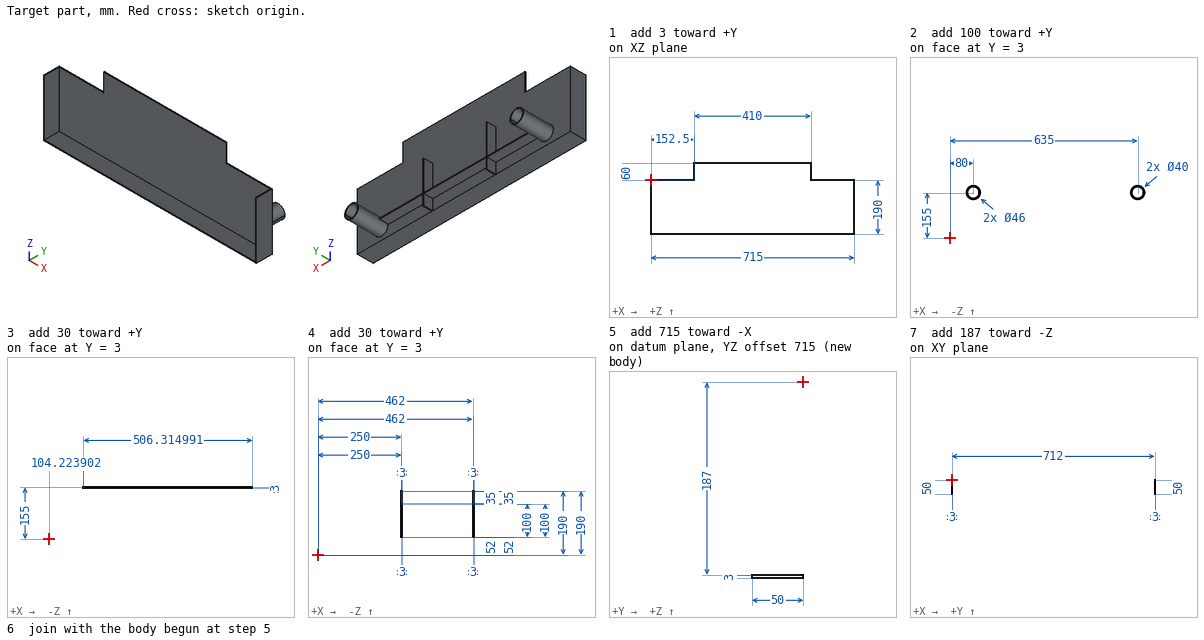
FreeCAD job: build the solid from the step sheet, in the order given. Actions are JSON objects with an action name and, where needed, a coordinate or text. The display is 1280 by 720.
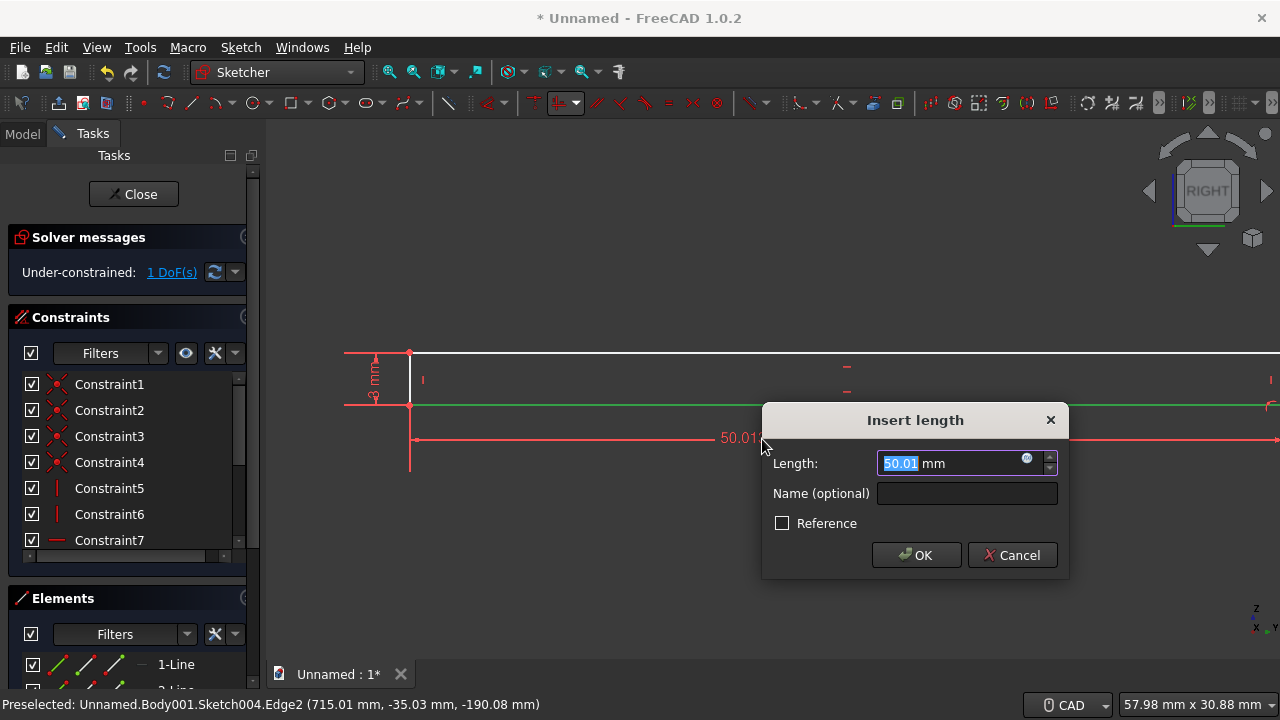
{"action": "type", "text": "50"}
{"action": "key", "text": "Return"}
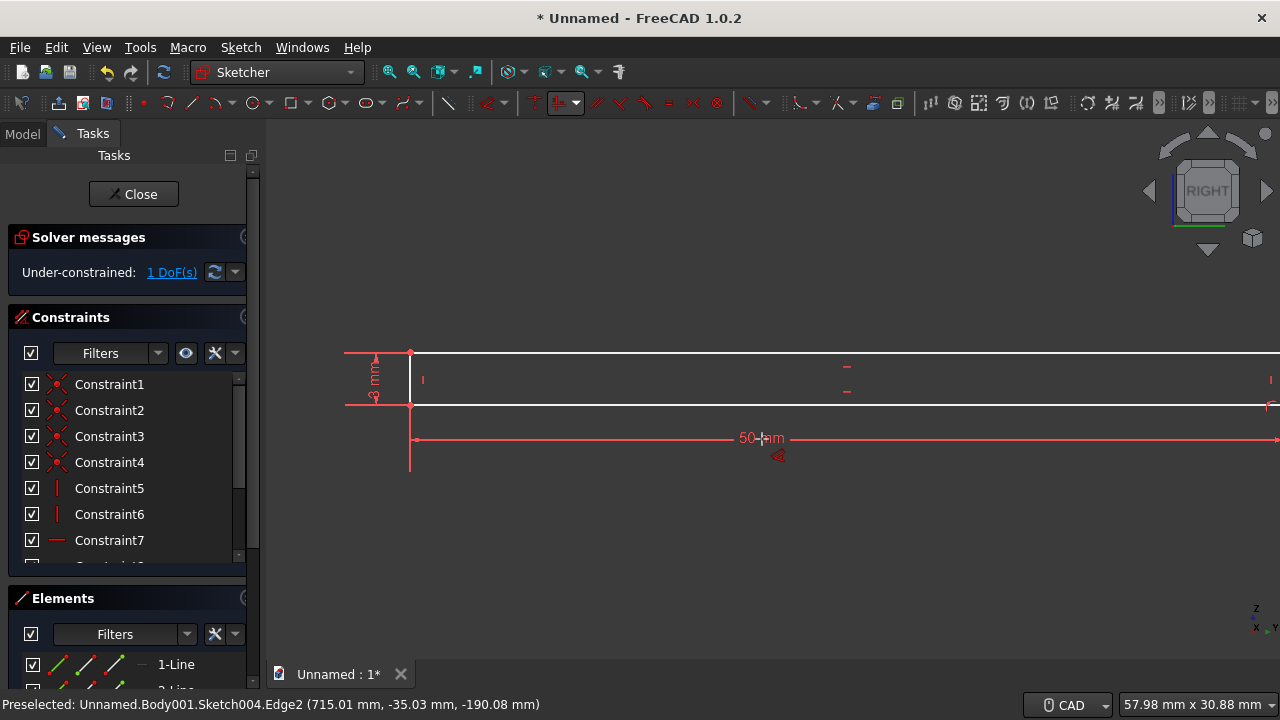
{"action": "left_click", "coordinate": [410, 353]}
{"action": "left_click", "coordinate": [376, 250]}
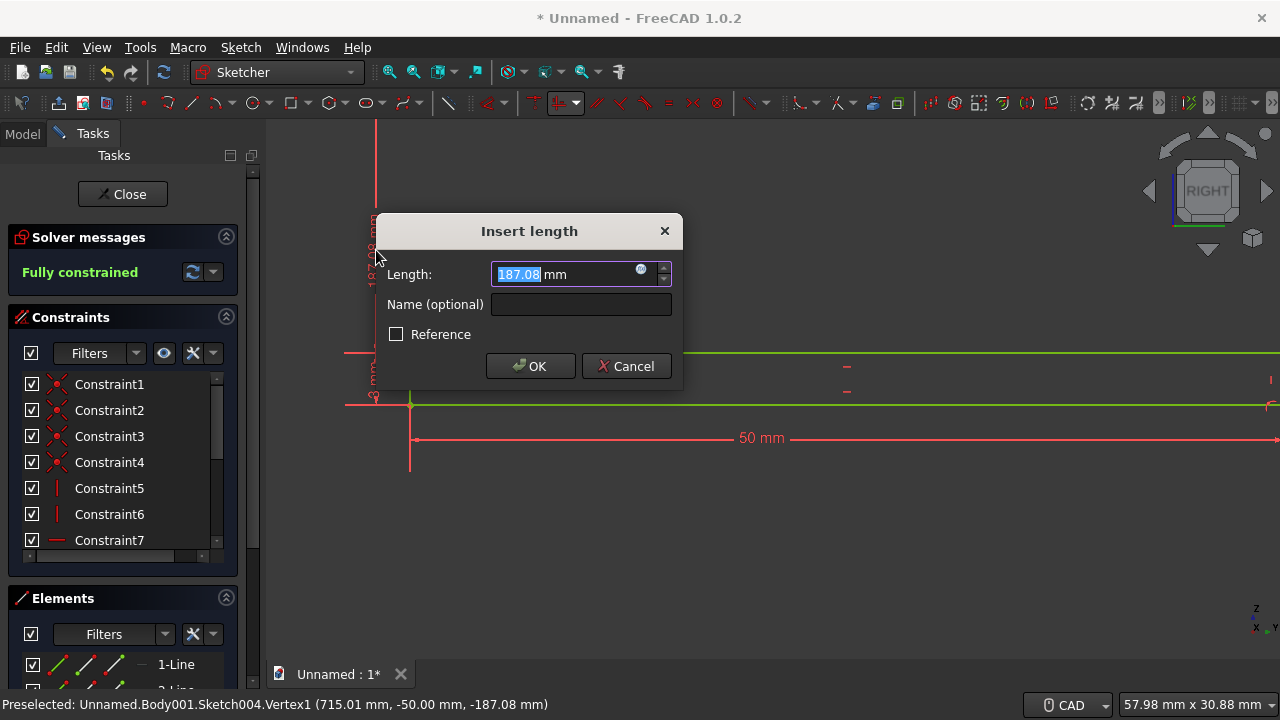
{"action": "type", "text": "187"}
{"action": "key", "text": "Return"}
{"action": "key", "text": "Escape"}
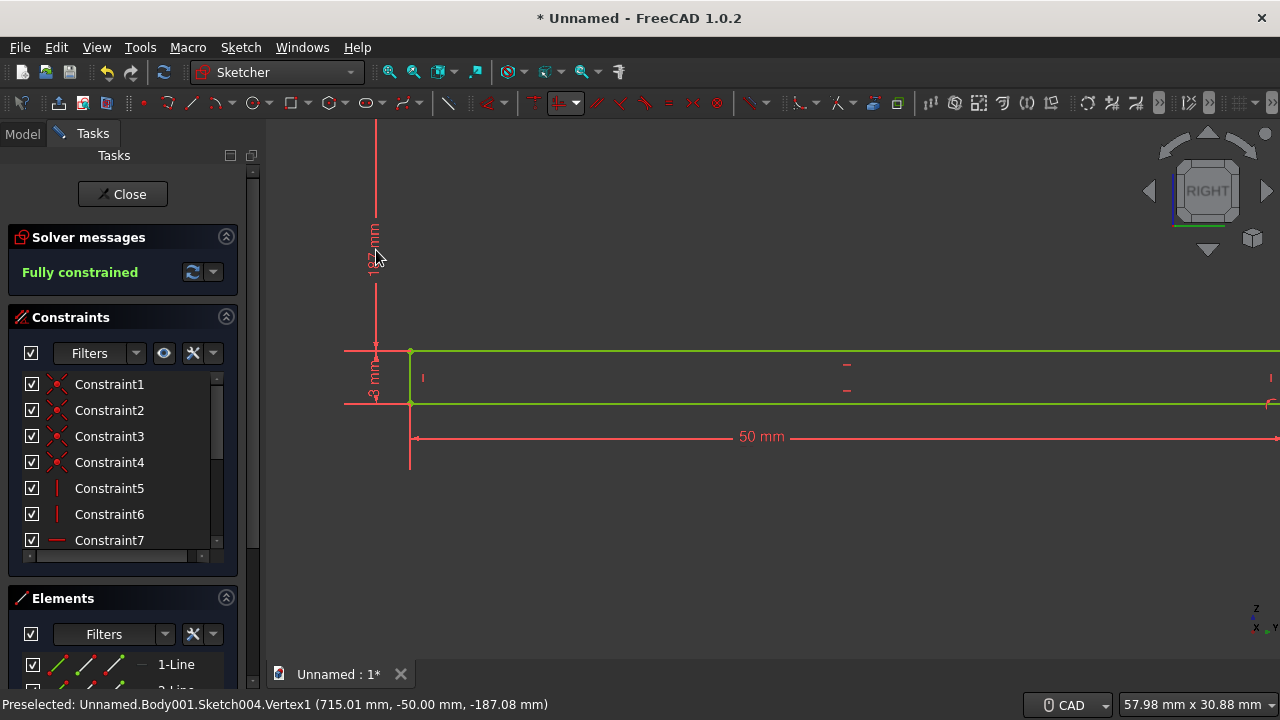
{"action": "left_click", "coordinate": [123, 194]}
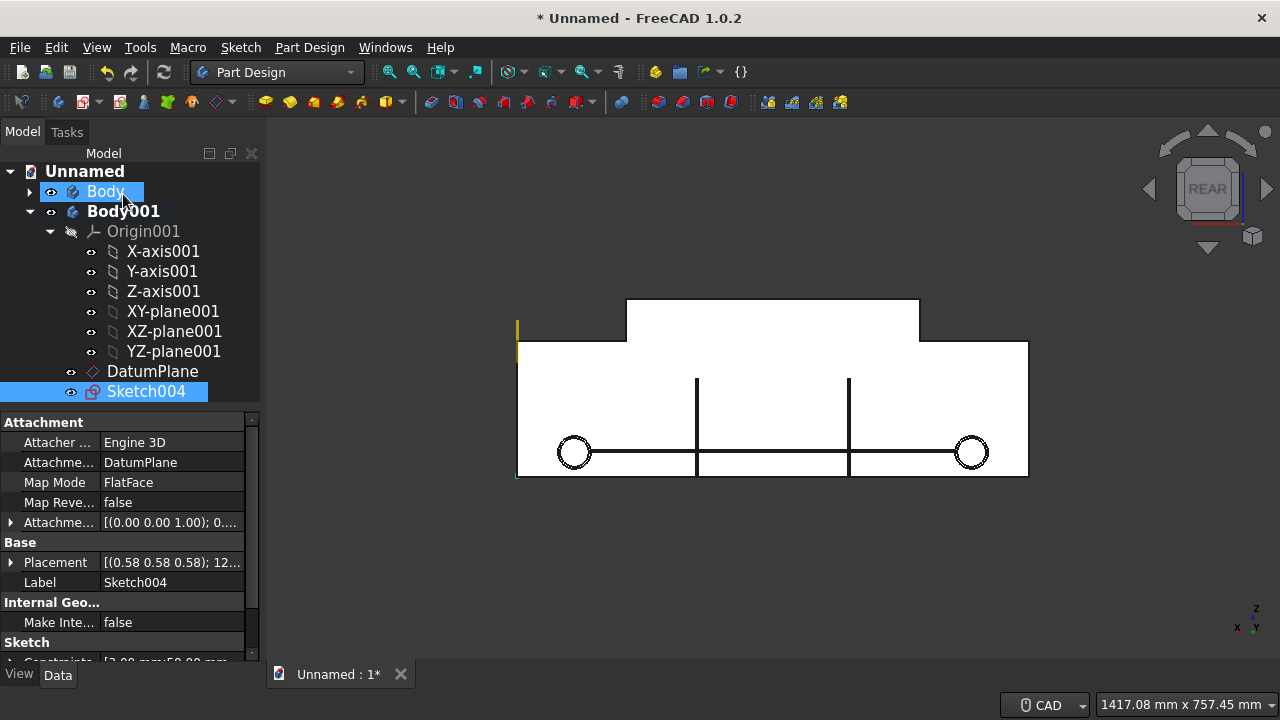
{"action": "left_click", "coordinate": [266, 102]}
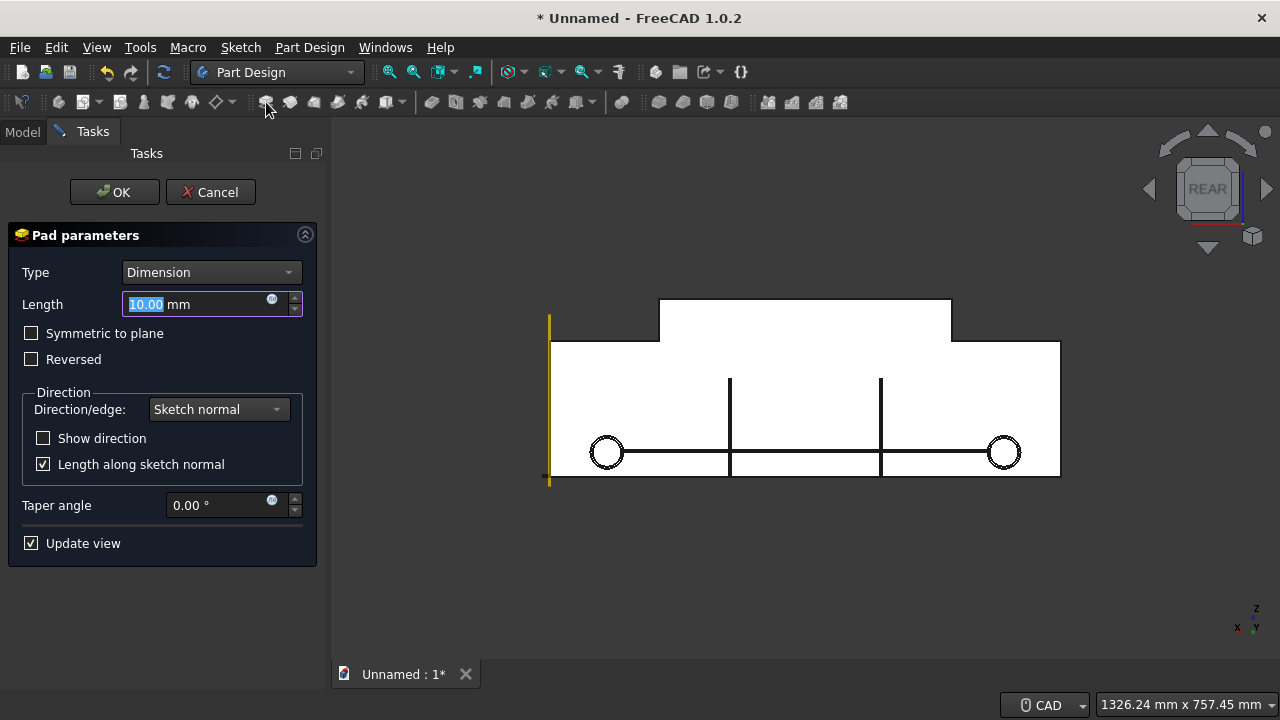
{"action": "type", "text": "715"}
{"action": "key", "text": "Tab"}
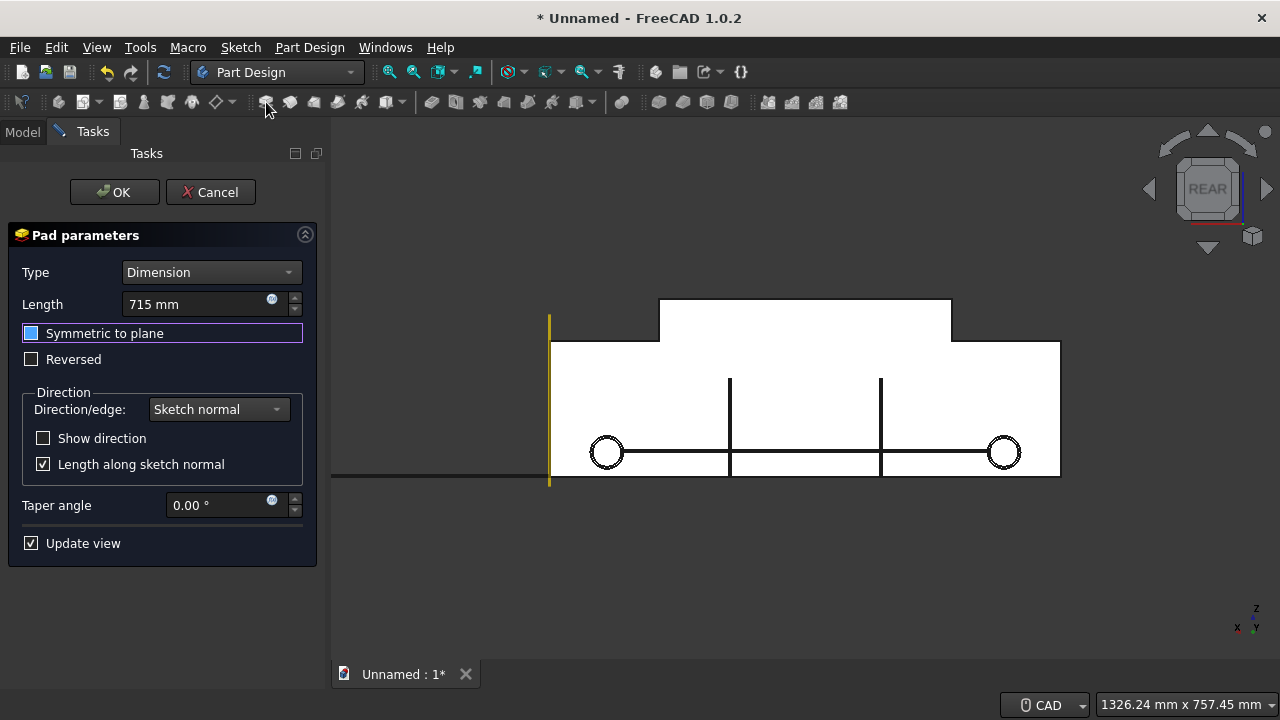
{"action": "left_click", "coordinate": [30, 359]}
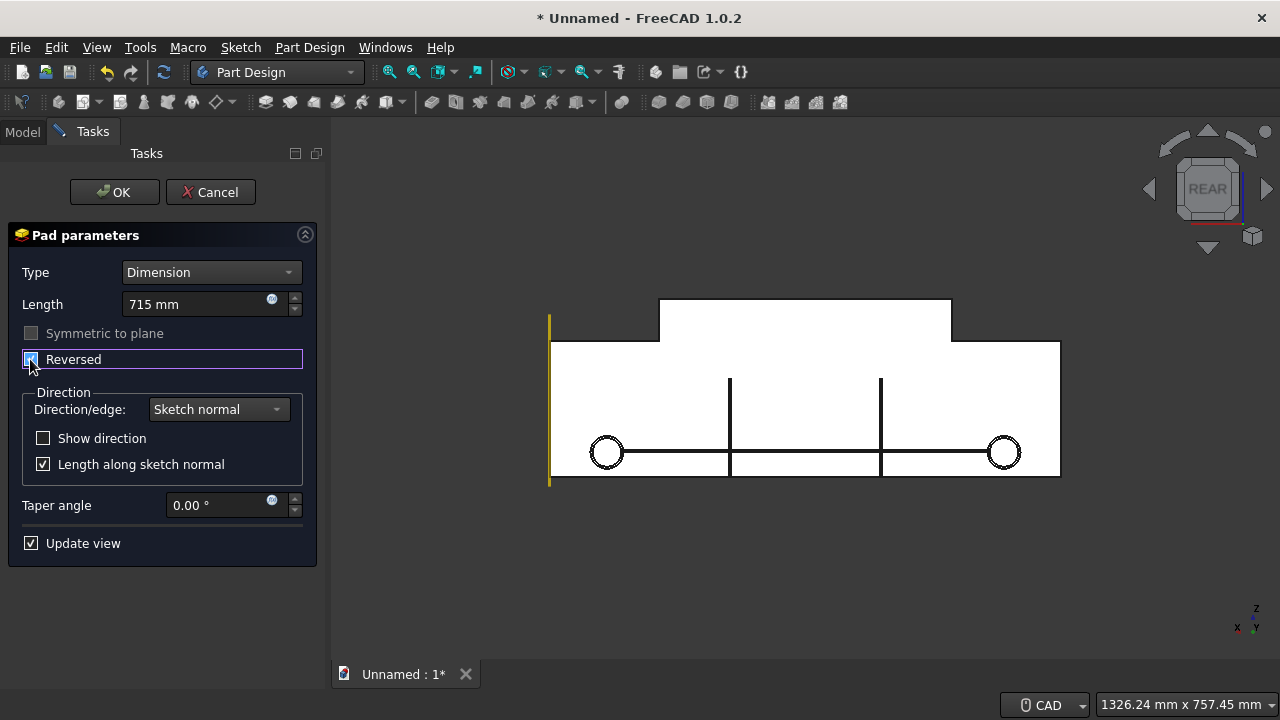
{"action": "left_click", "coordinate": [115, 192]}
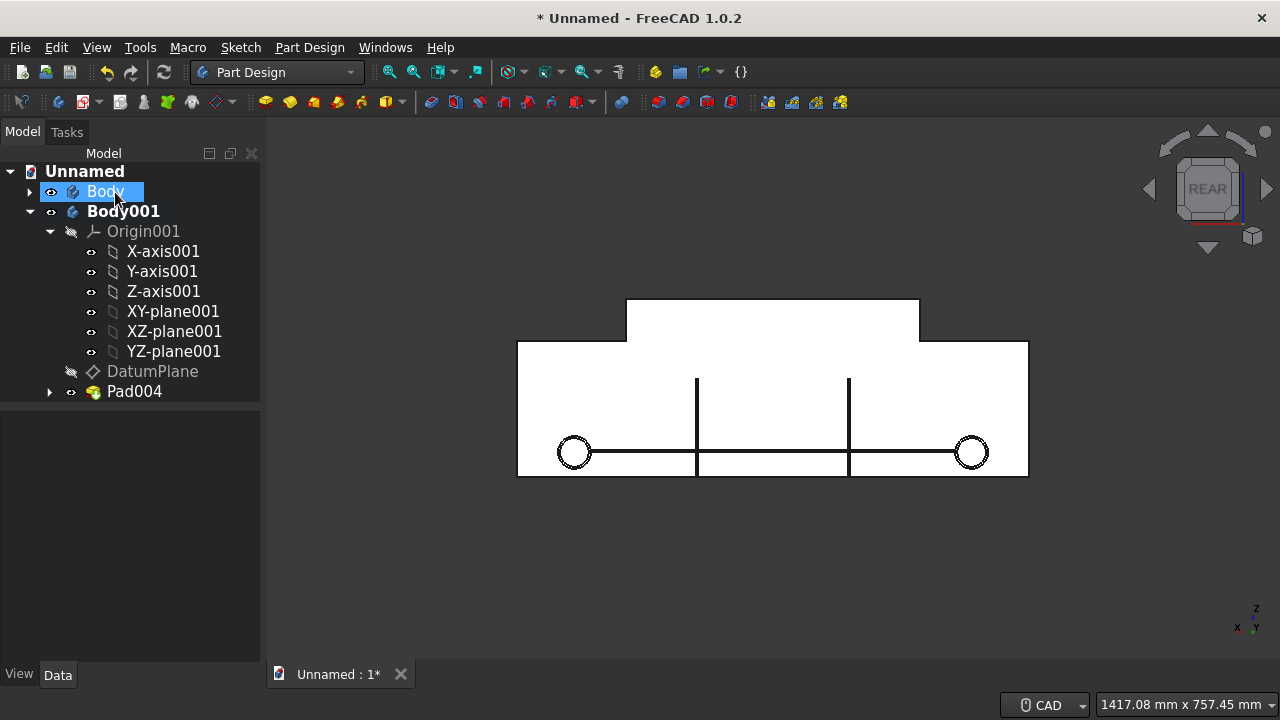
{"action": "double_click", "coordinate": [96, 192]}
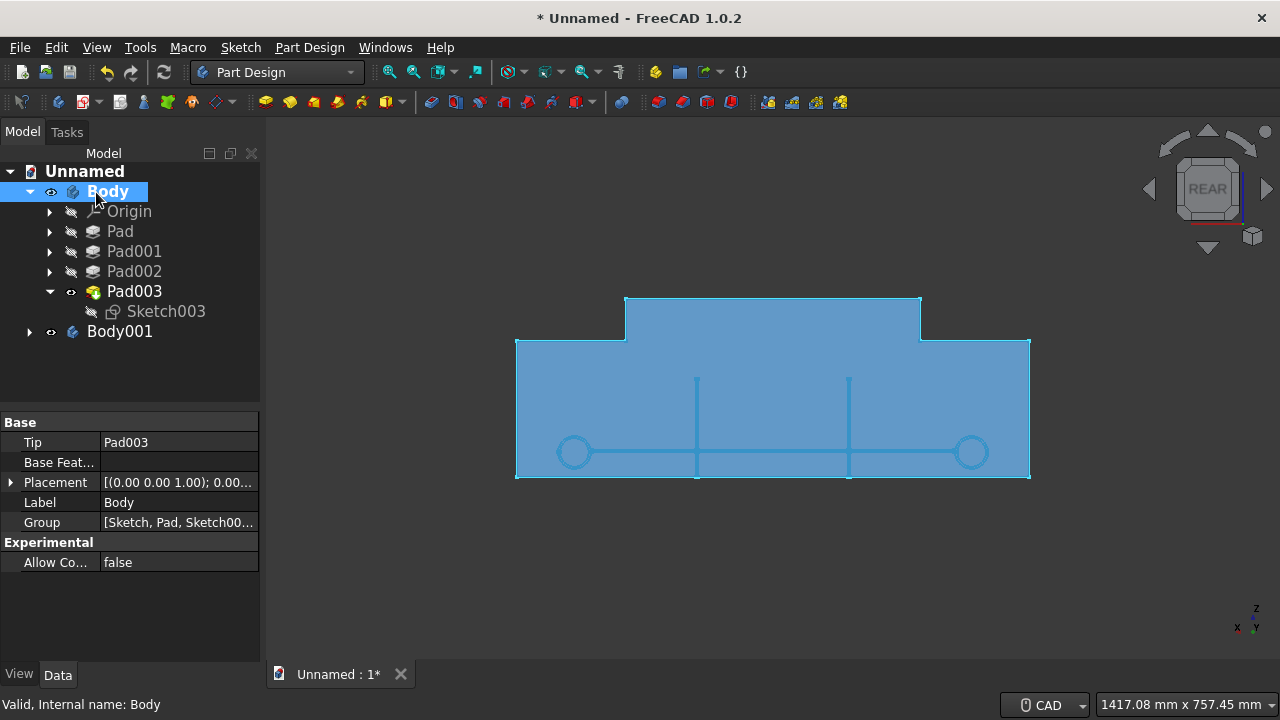
{"action": "left_click", "coordinate": [96, 332]}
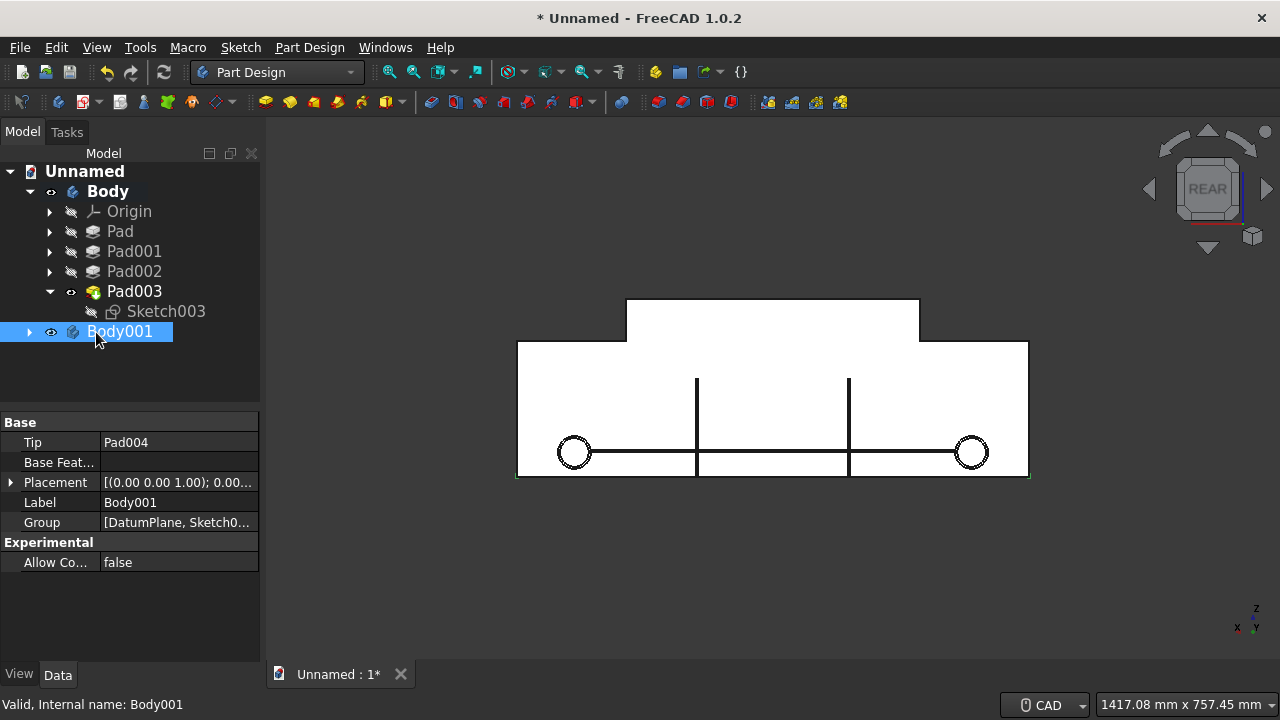
{"action": "left_click", "coordinate": [622, 102]}